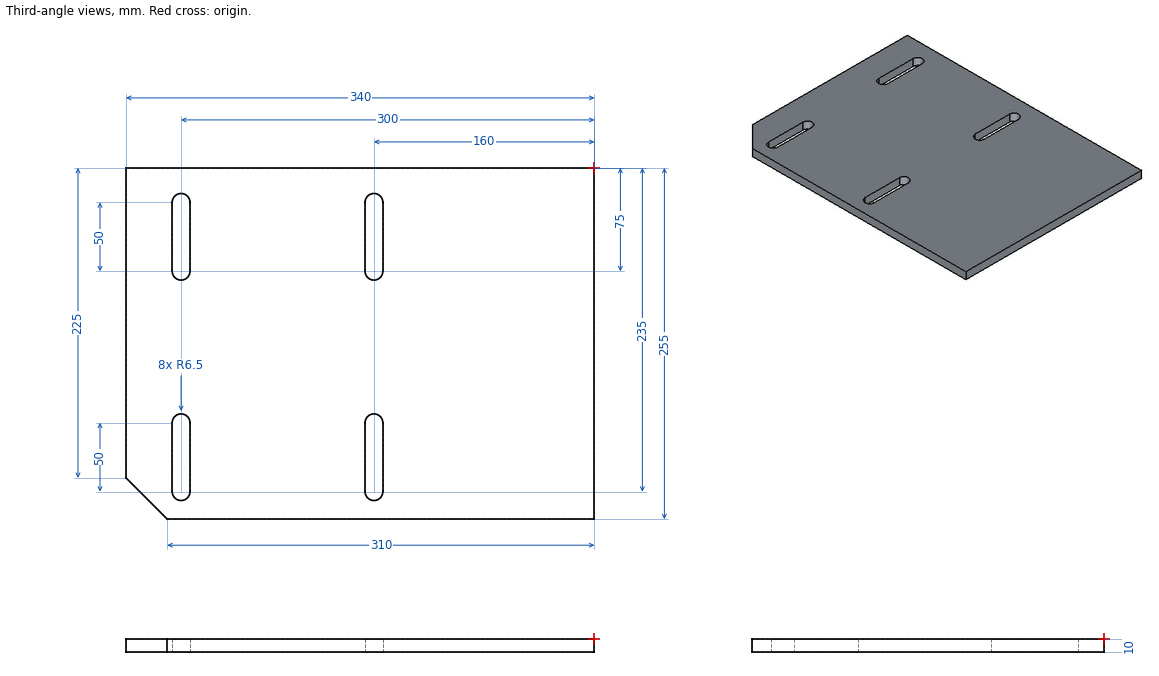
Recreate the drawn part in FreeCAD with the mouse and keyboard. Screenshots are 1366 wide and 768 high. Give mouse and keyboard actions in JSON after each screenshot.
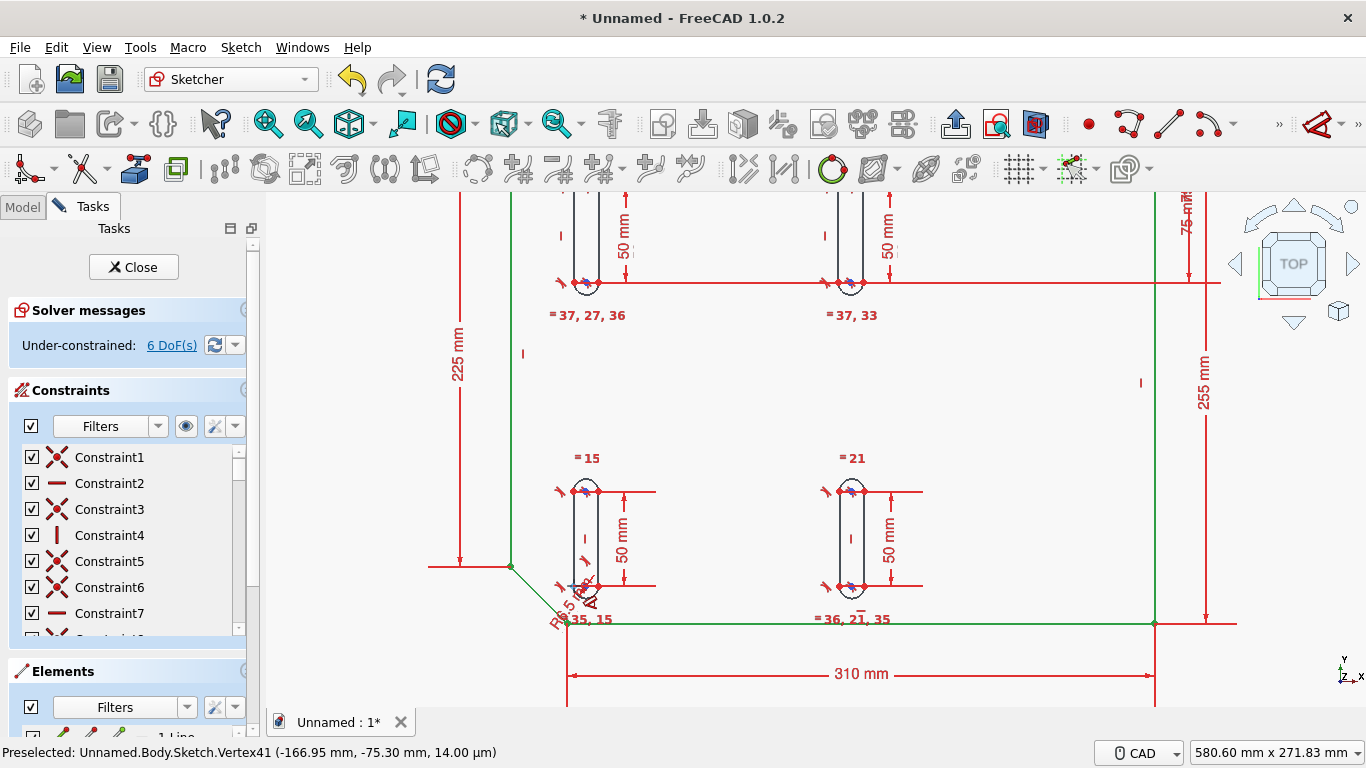
{"action": "left_click", "coordinate": [574, 586]}
{"action": "left_click", "coordinate": [1189, 403]}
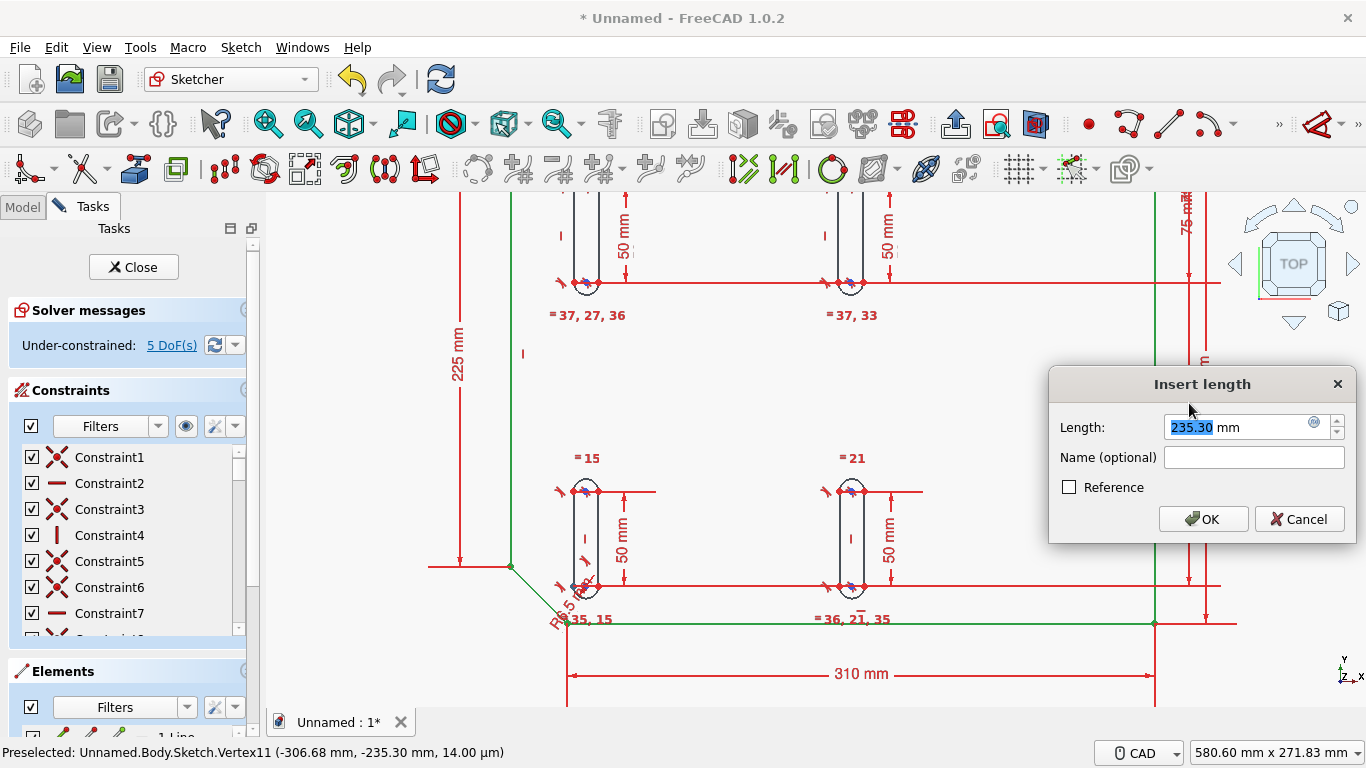
{"action": "type", "text": "235"}
{"action": "key", "text": "Return"}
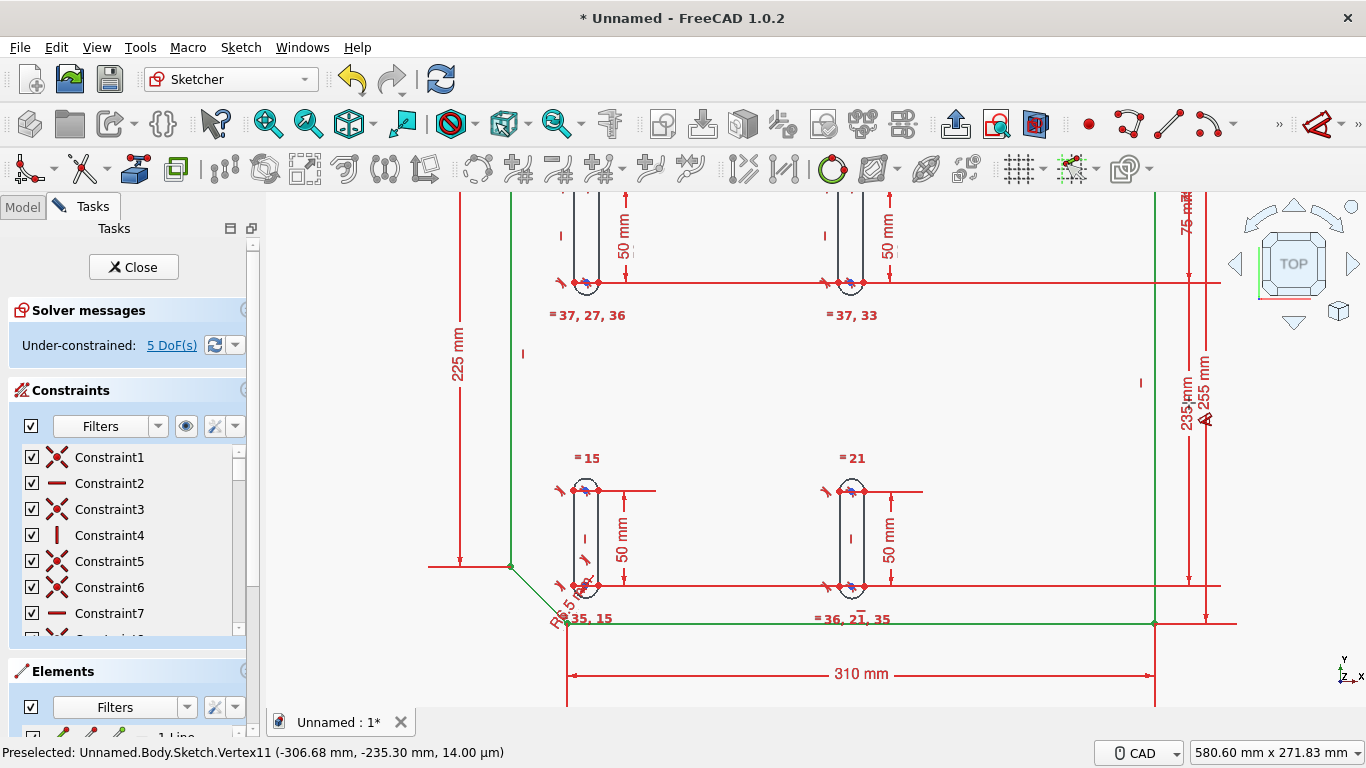
{"action": "left_click", "coordinate": [840, 586]}
{"action": "left_click", "coordinate": [1189, 319]}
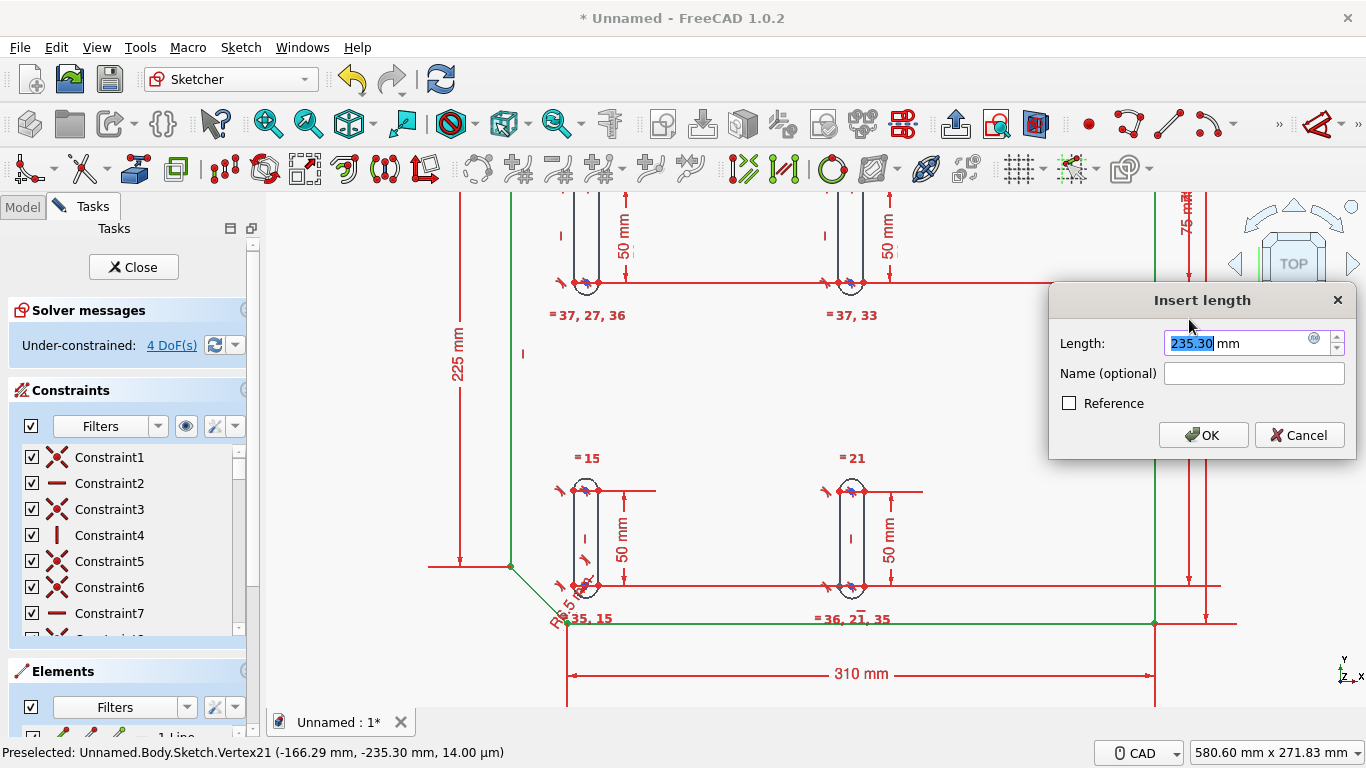
{"action": "type", "text": "235"}
{"action": "key", "text": "Return"}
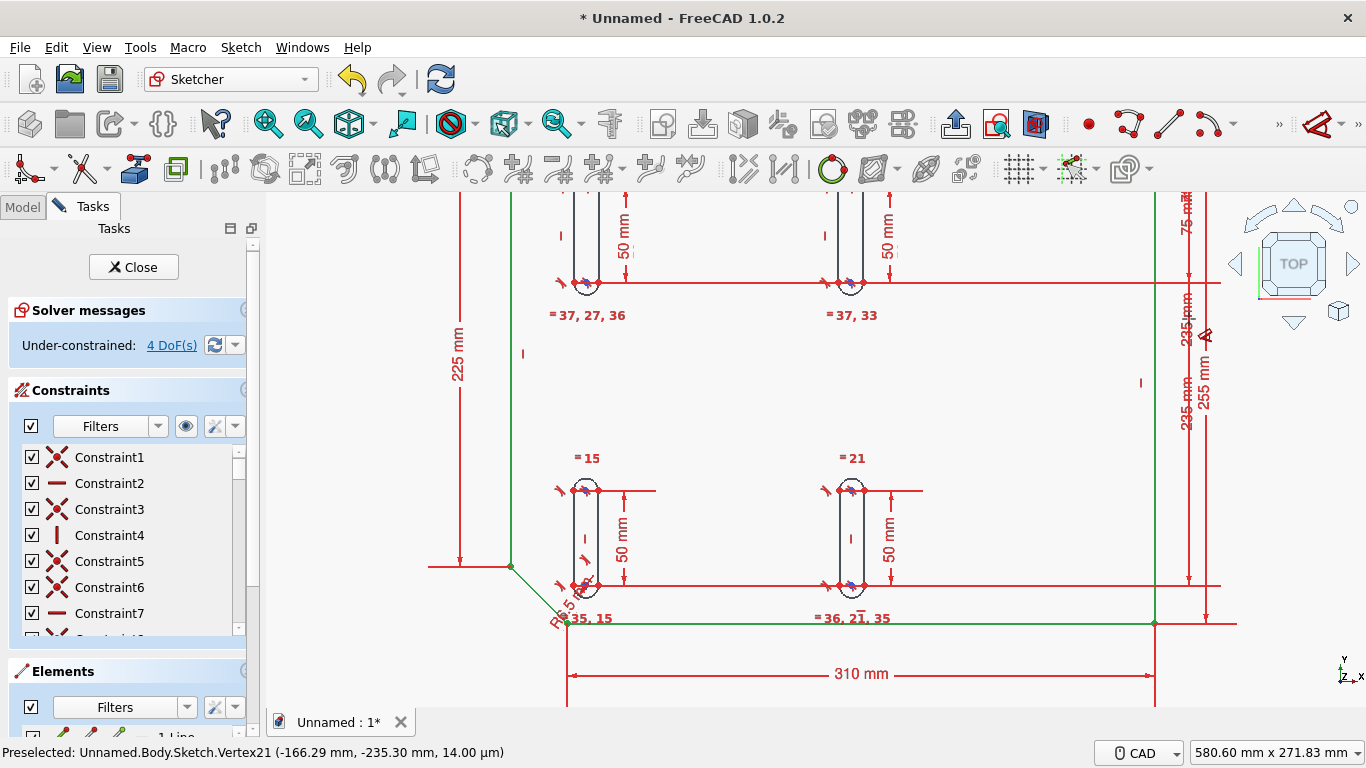
{"action": "left_click", "coordinate": [586, 586]}
{"action": "left_click", "coordinate": [870, 644]}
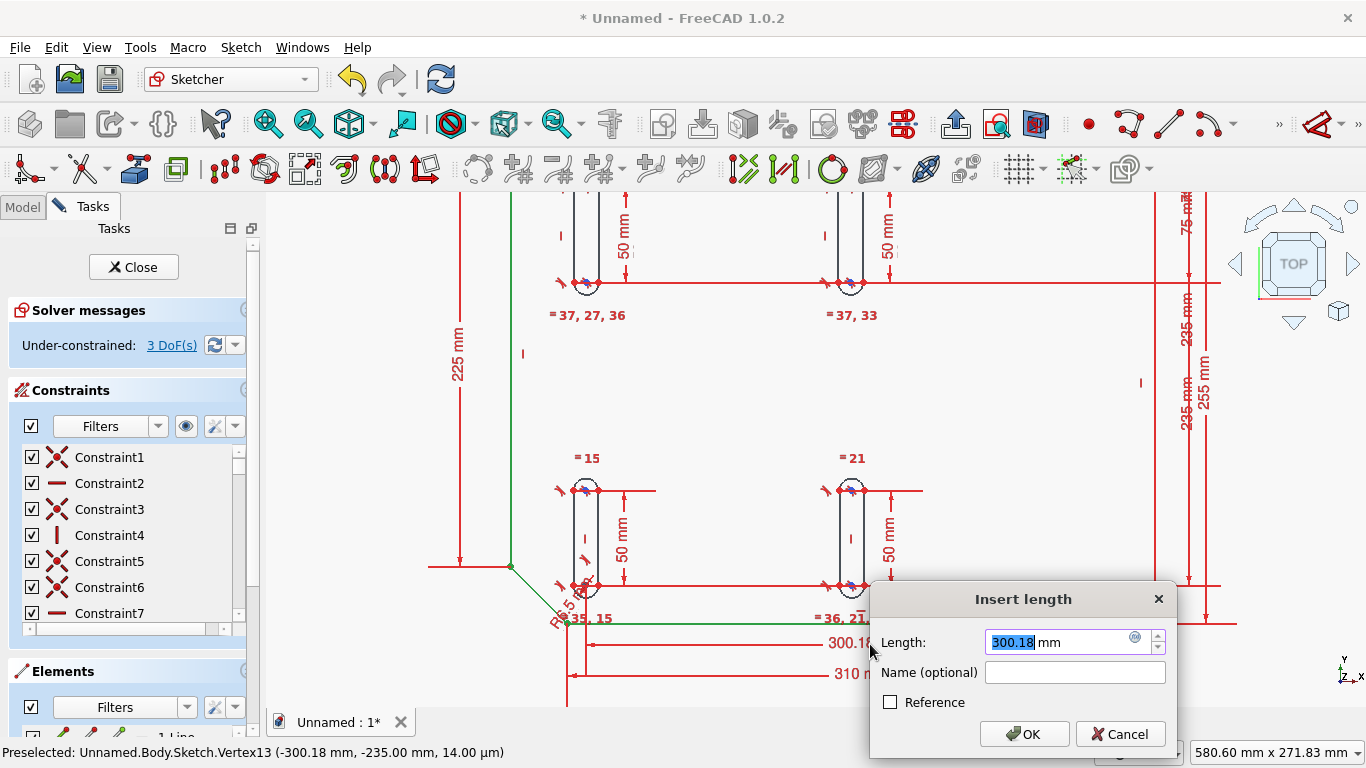
{"action": "type", "text": "300"}
{"action": "key", "text": "Return"}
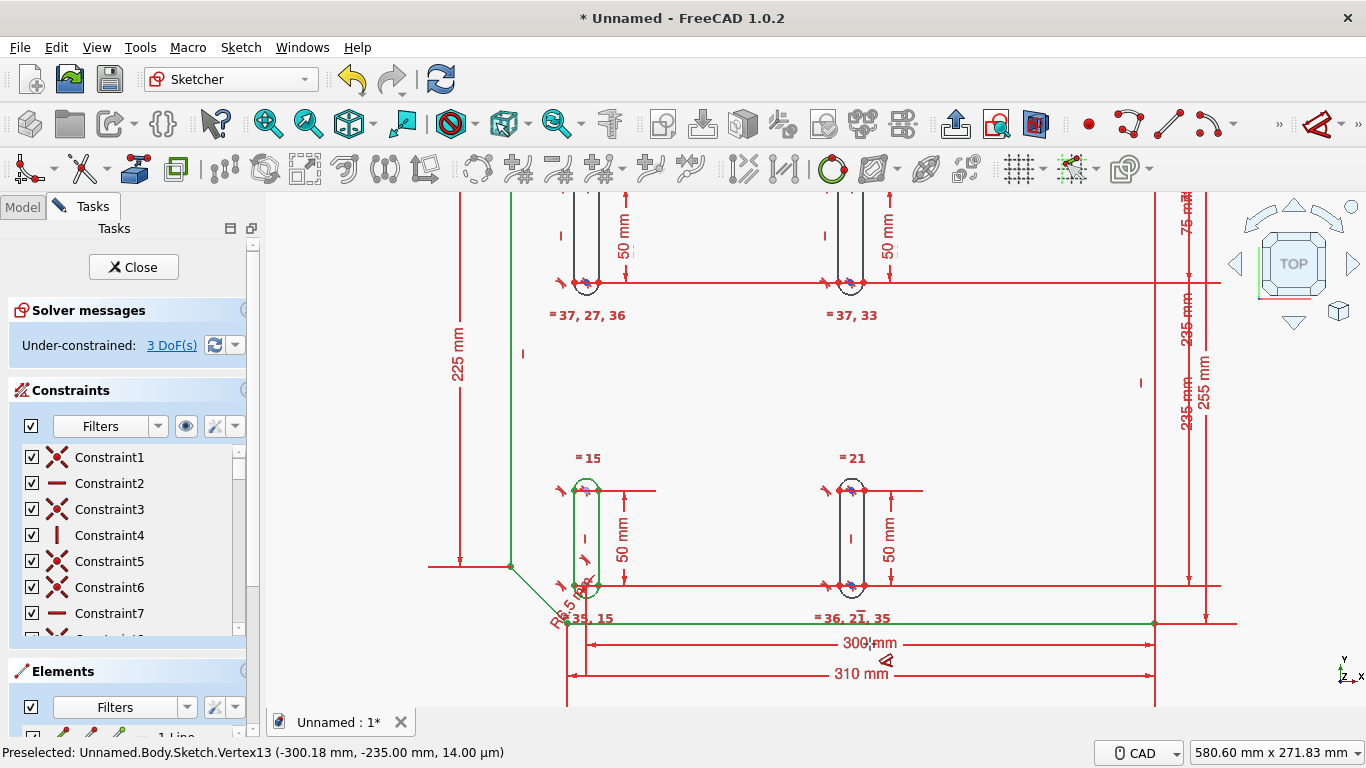
{"action": "left_click", "coordinate": [852, 586]}
{"action": "left_click", "coordinate": [1003, 644]}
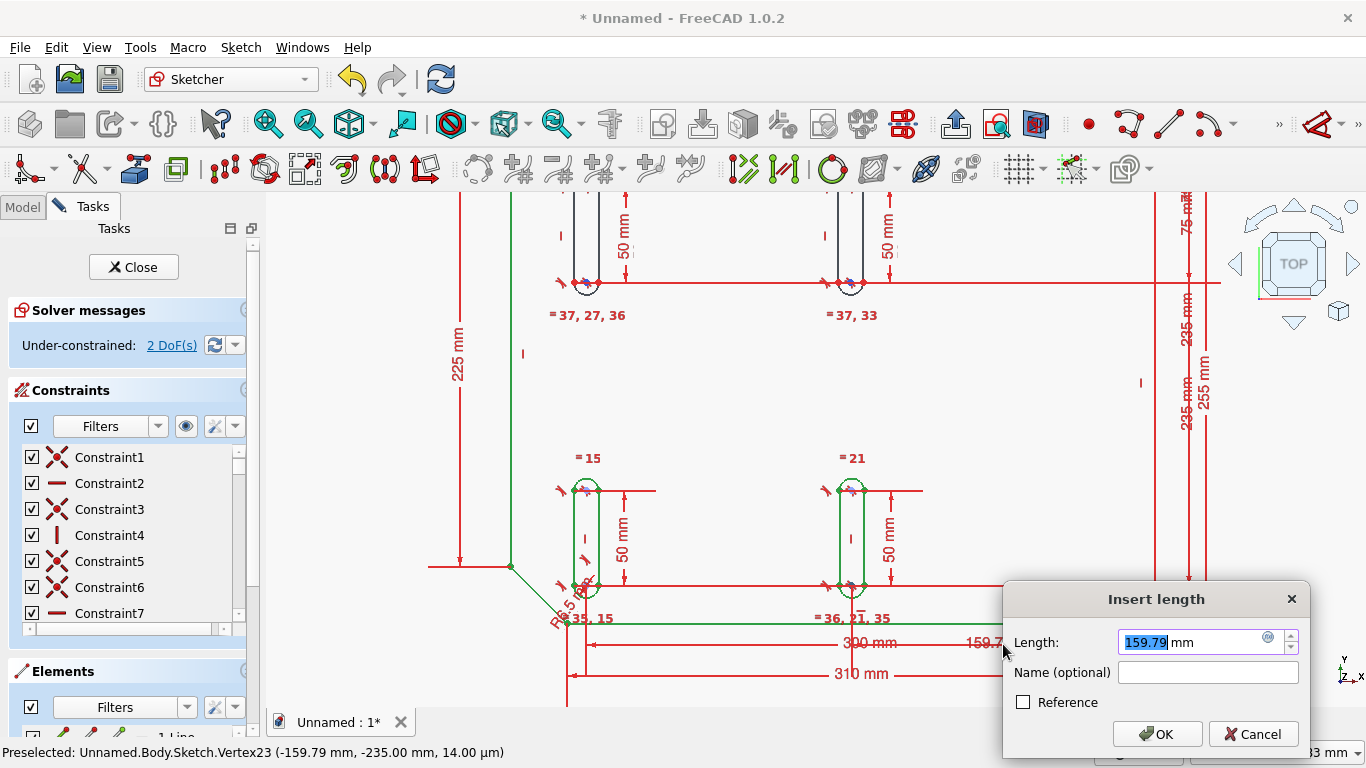
{"action": "type", "text": "160"}
{"action": "key", "text": "Return"}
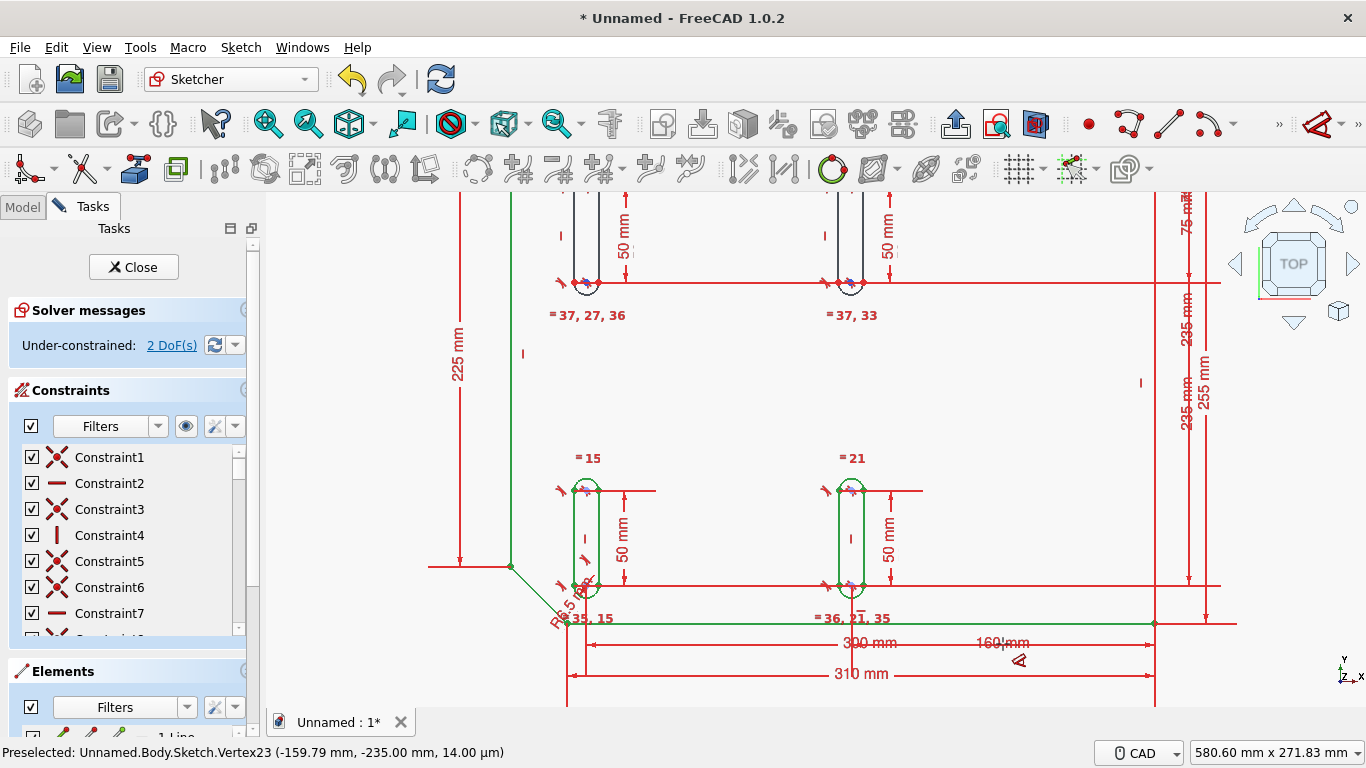
{"action": "left_click", "coordinate": [587, 283]}
{"action": "left_click", "coordinate": [871, 317]}